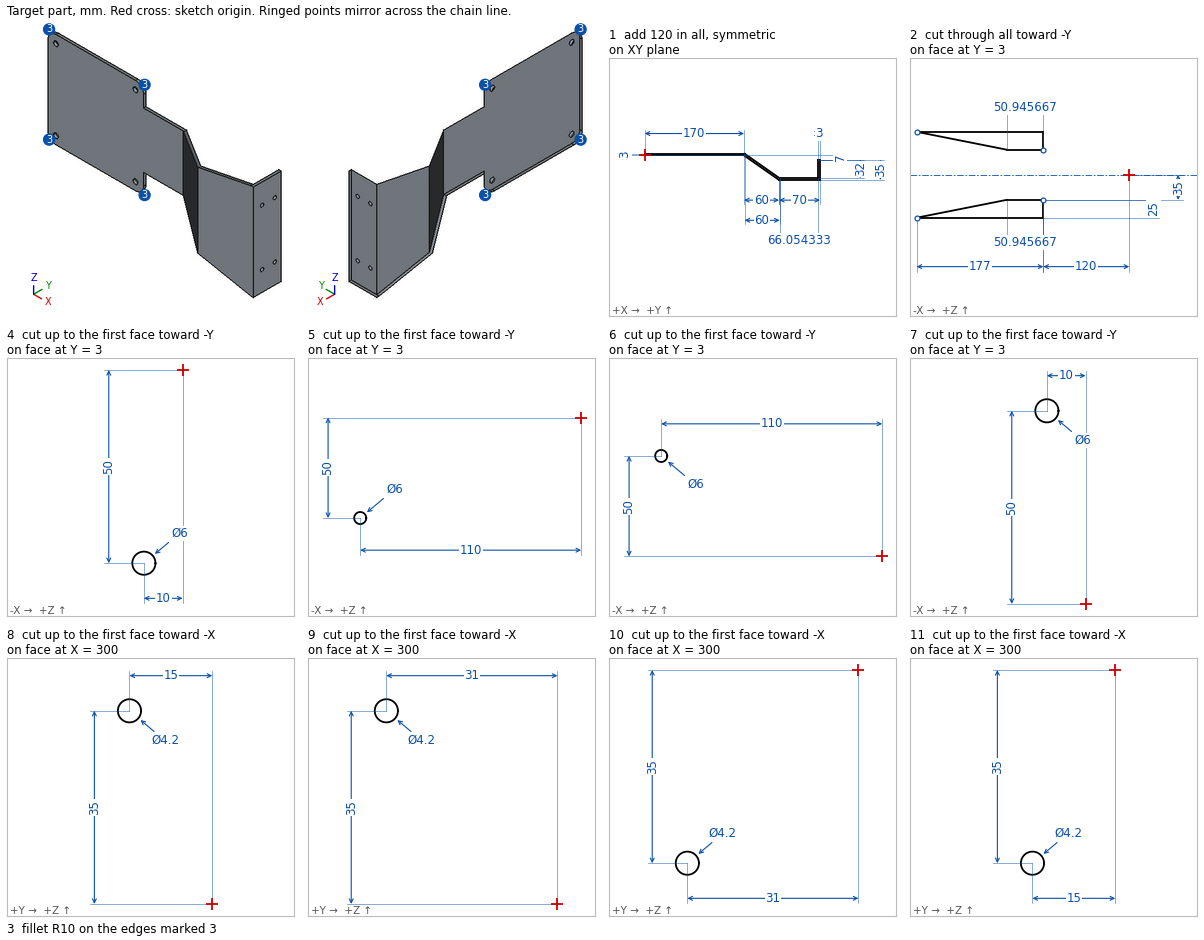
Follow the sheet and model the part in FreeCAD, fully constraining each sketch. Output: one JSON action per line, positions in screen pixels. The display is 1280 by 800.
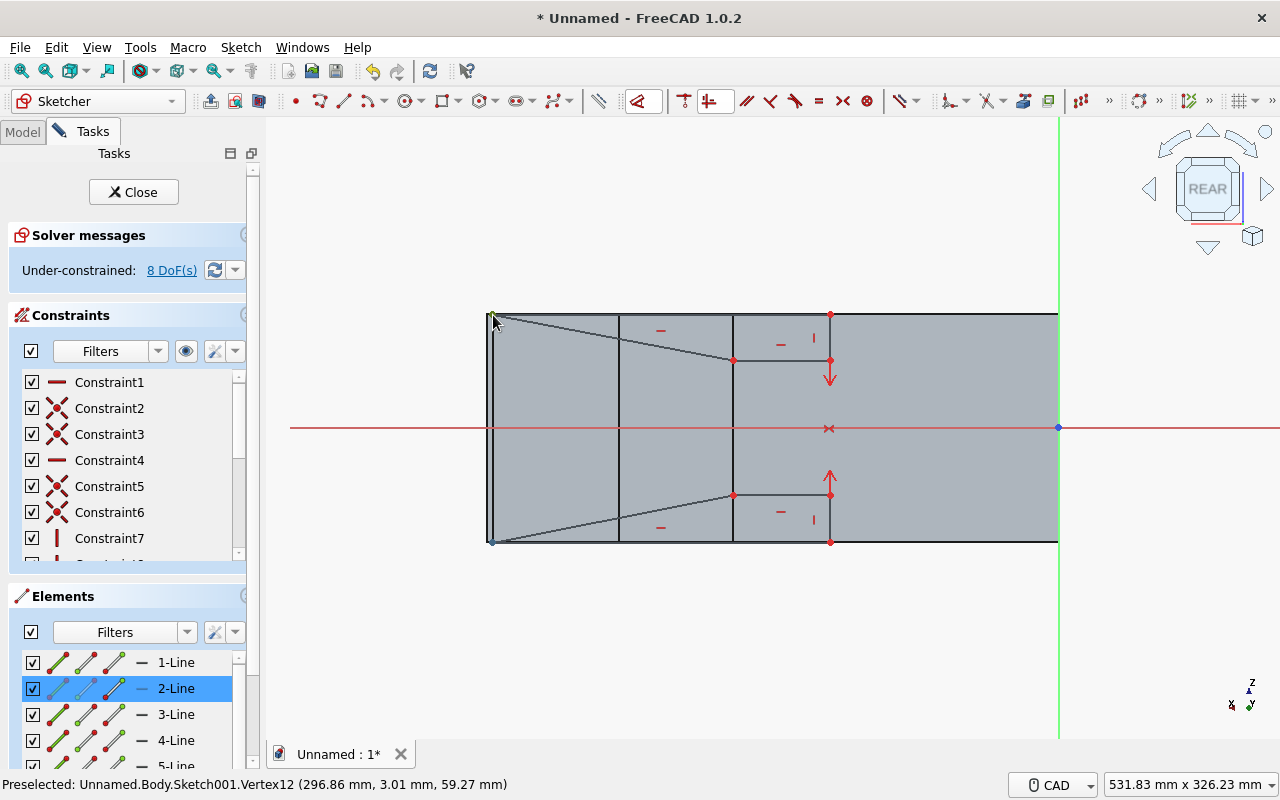
{"action": "left_click", "coordinate": [353, 428]}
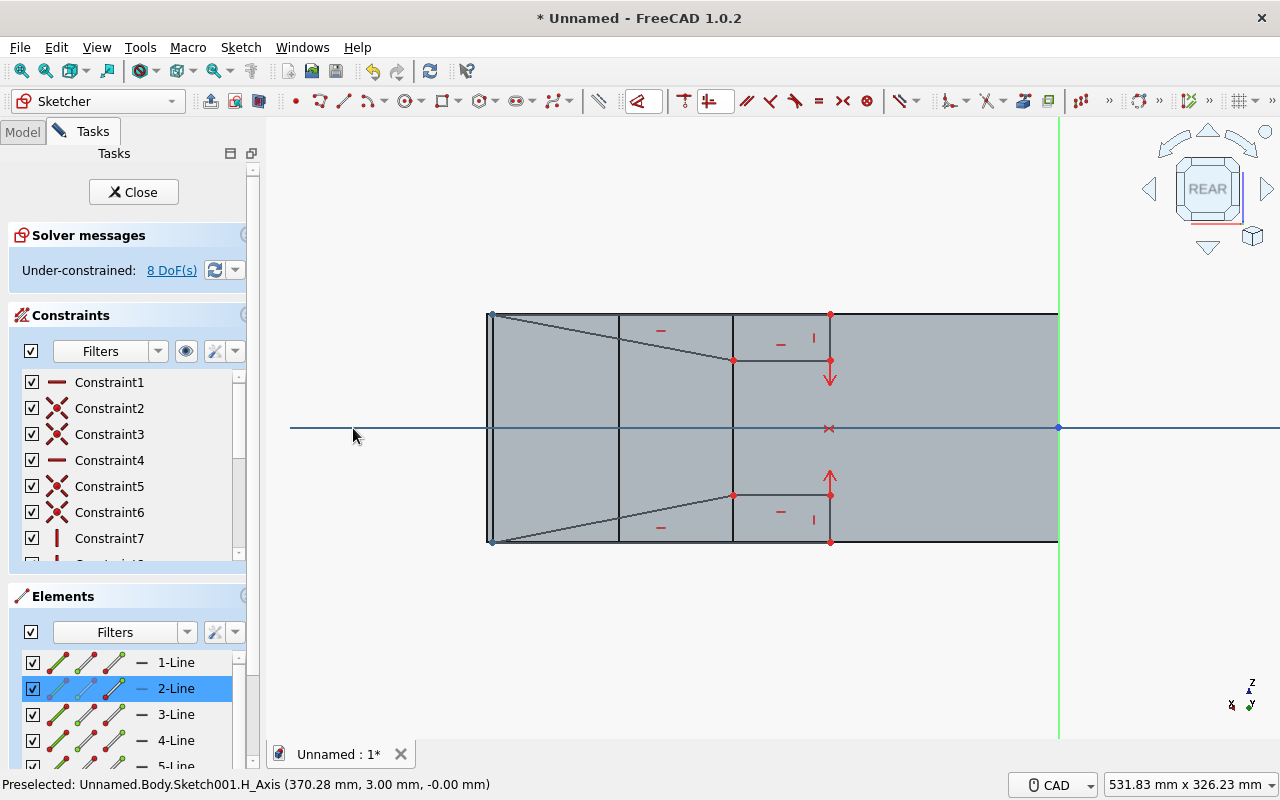
{"action": "left_click", "coordinate": [844, 102]}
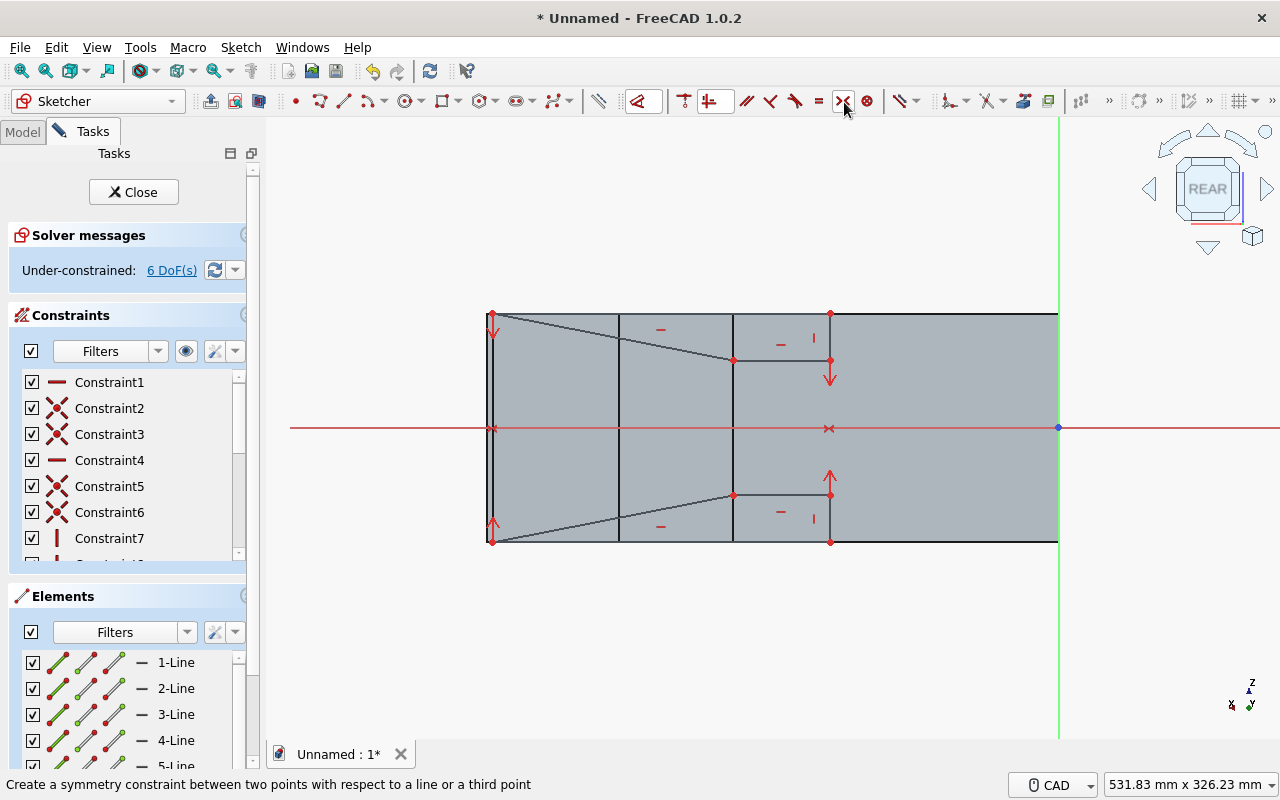
{"action": "left_click", "coordinate": [830, 528]}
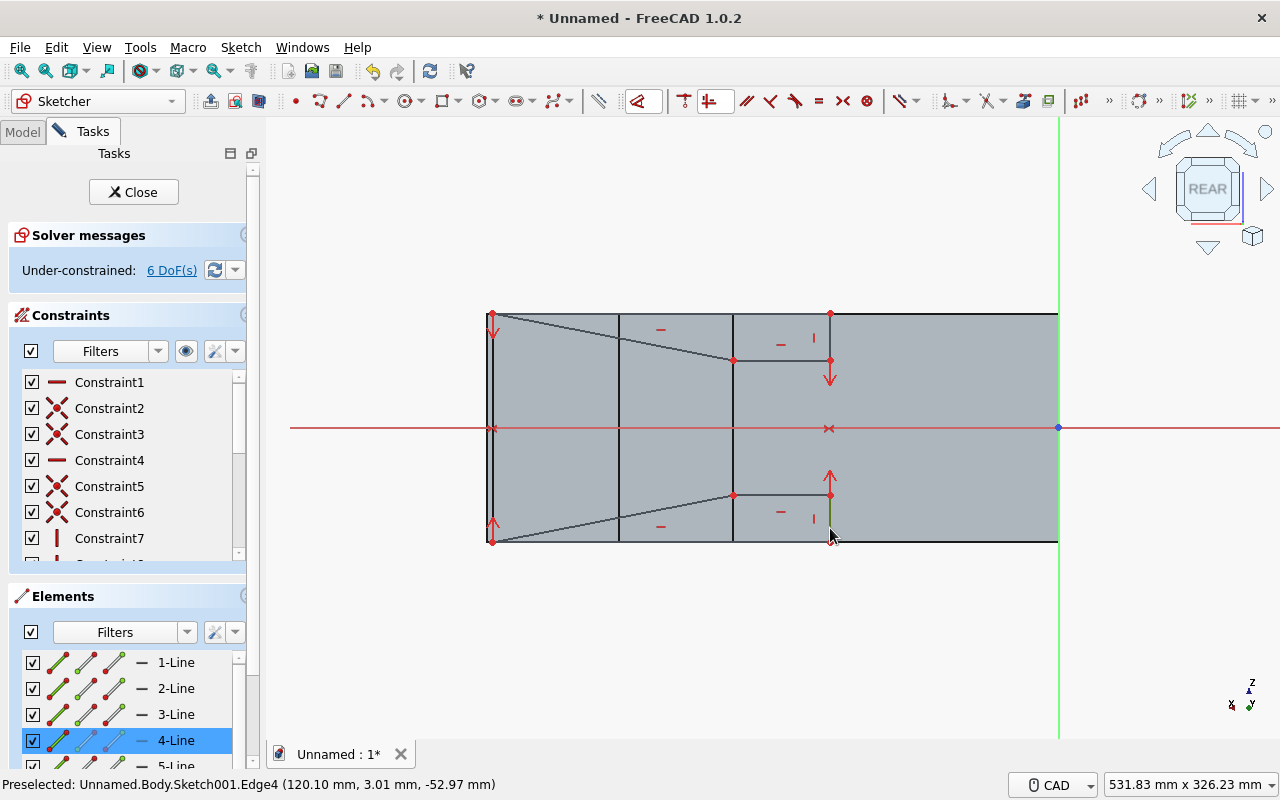
{"action": "left_click", "coordinate": [656, 102]}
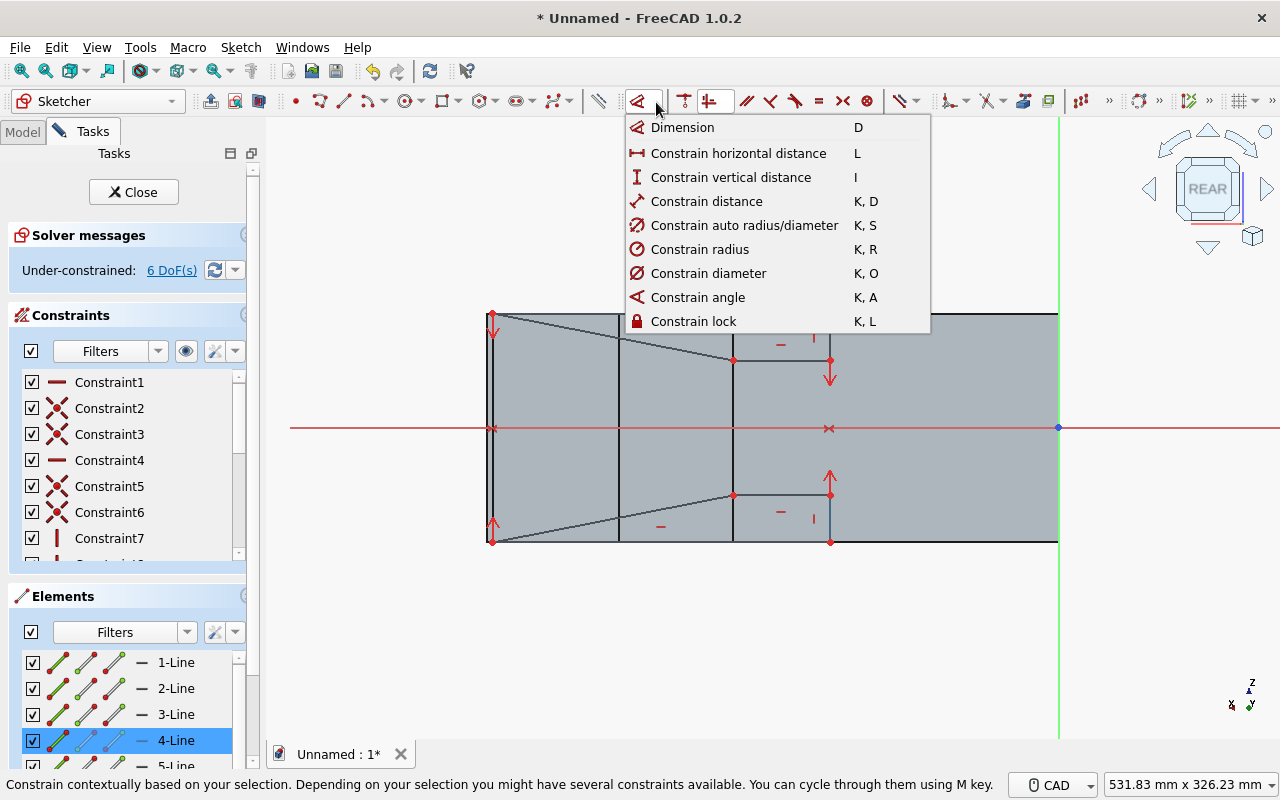
{"action": "left_click", "coordinate": [778, 177]}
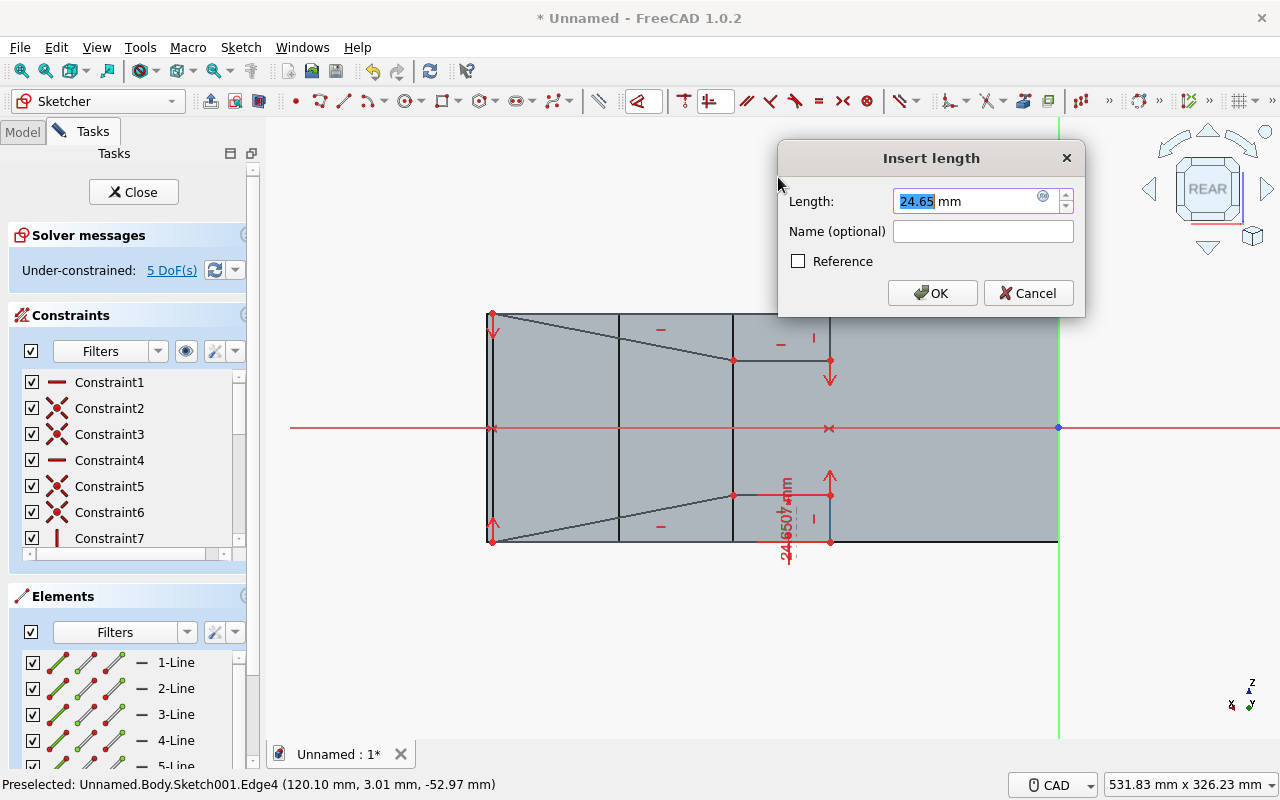
{"action": "type", "text": "25"}
{"action": "key", "text": "Return"}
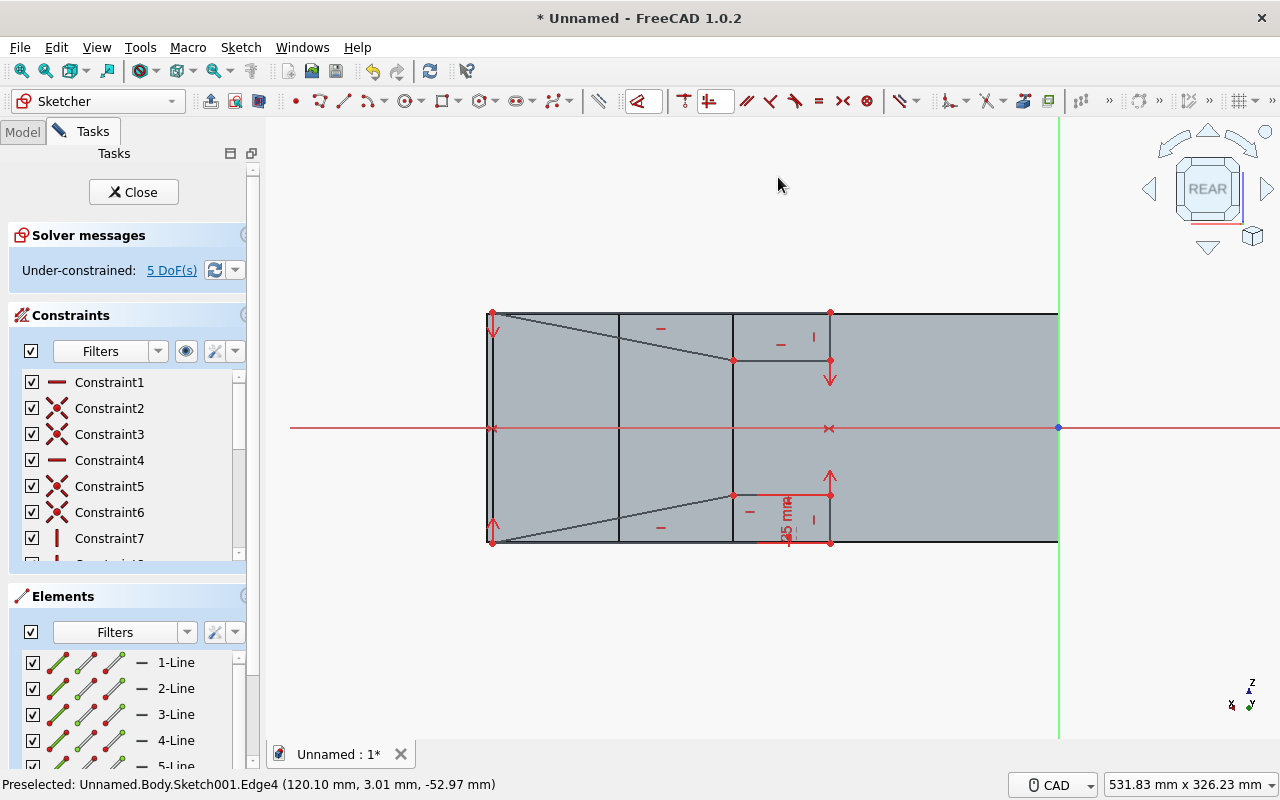
{"action": "left_click", "coordinate": [594, 543]}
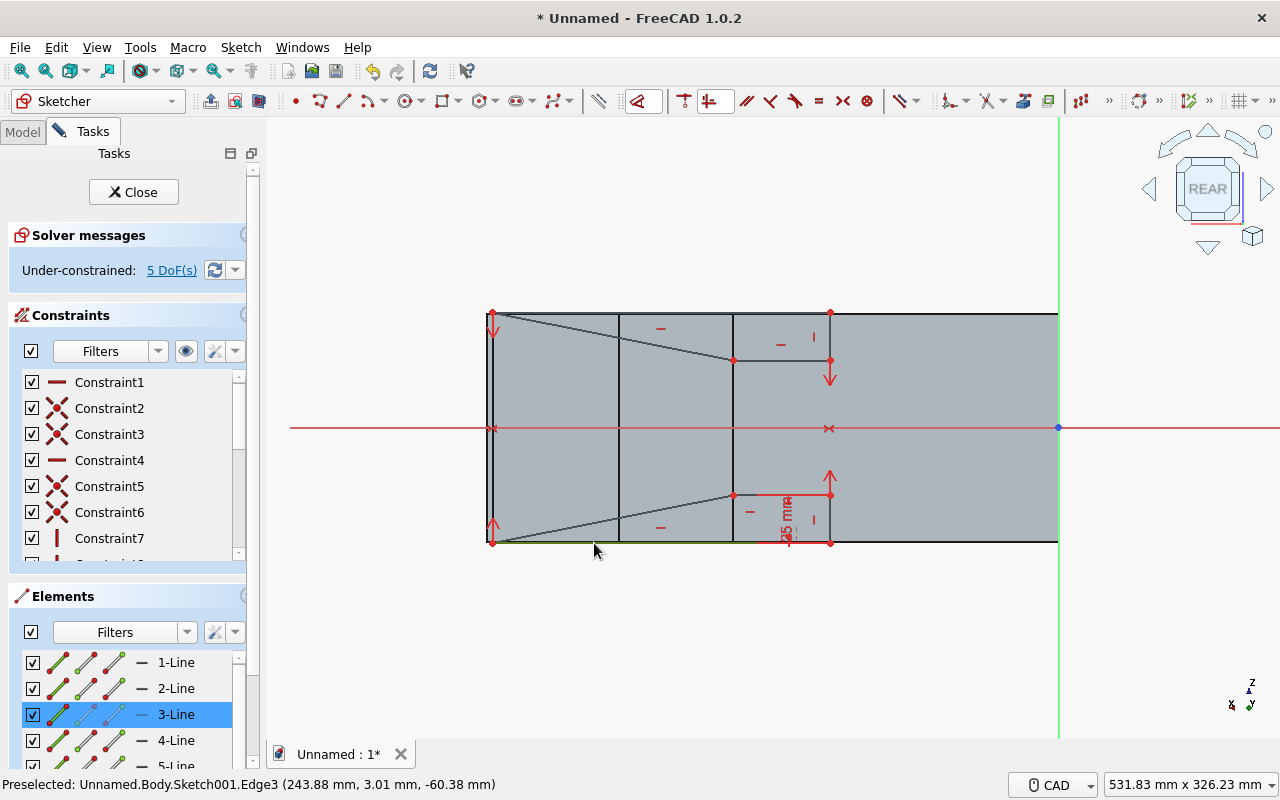
{"action": "left_click", "coordinate": [656, 102]}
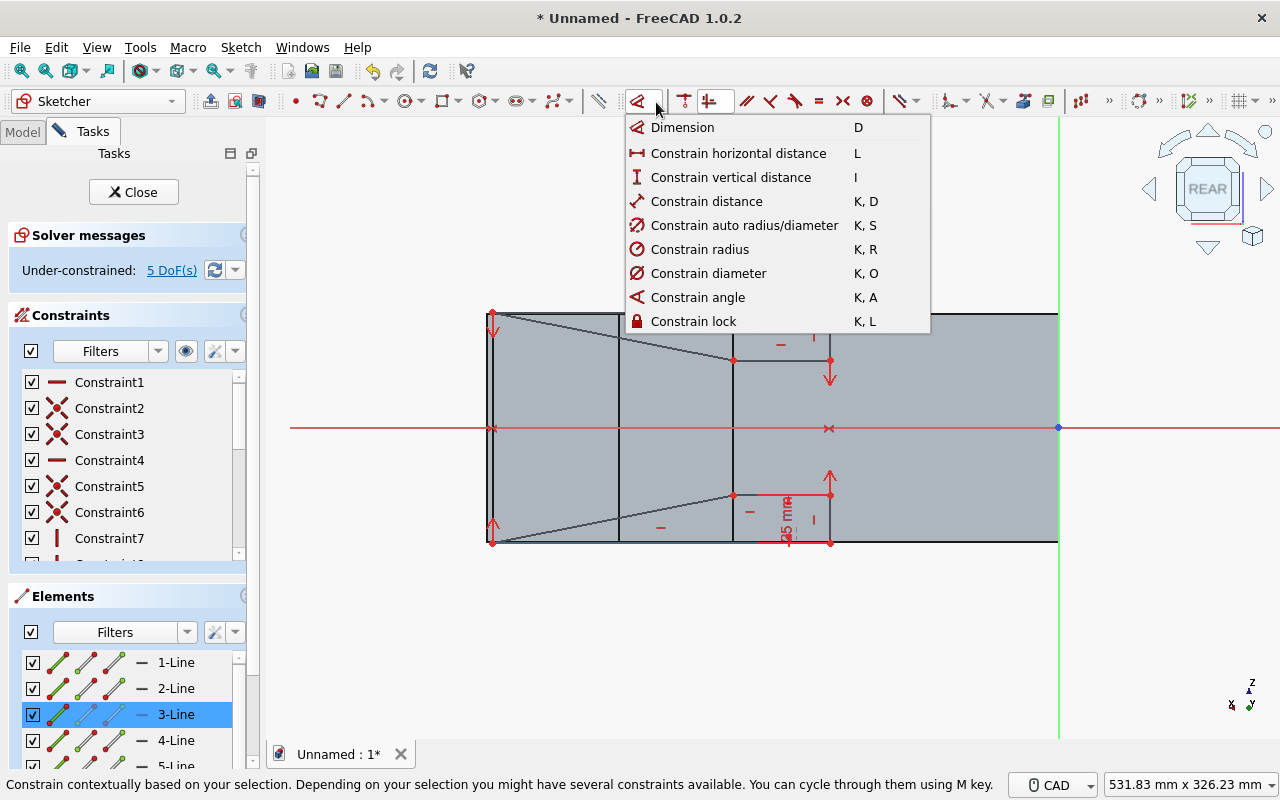
{"action": "left_click", "coordinate": [778, 153]}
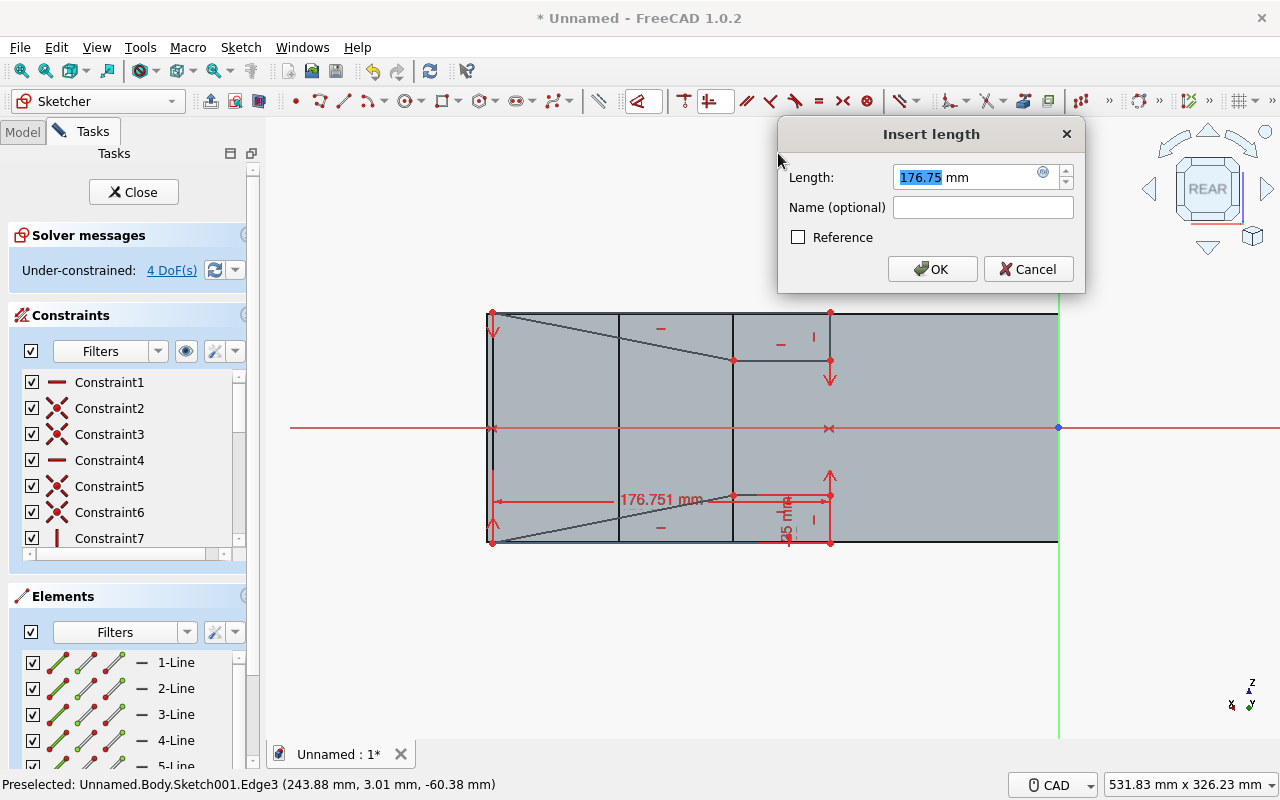
{"action": "type", "text": "177"}
{"action": "key", "text": "Return"}